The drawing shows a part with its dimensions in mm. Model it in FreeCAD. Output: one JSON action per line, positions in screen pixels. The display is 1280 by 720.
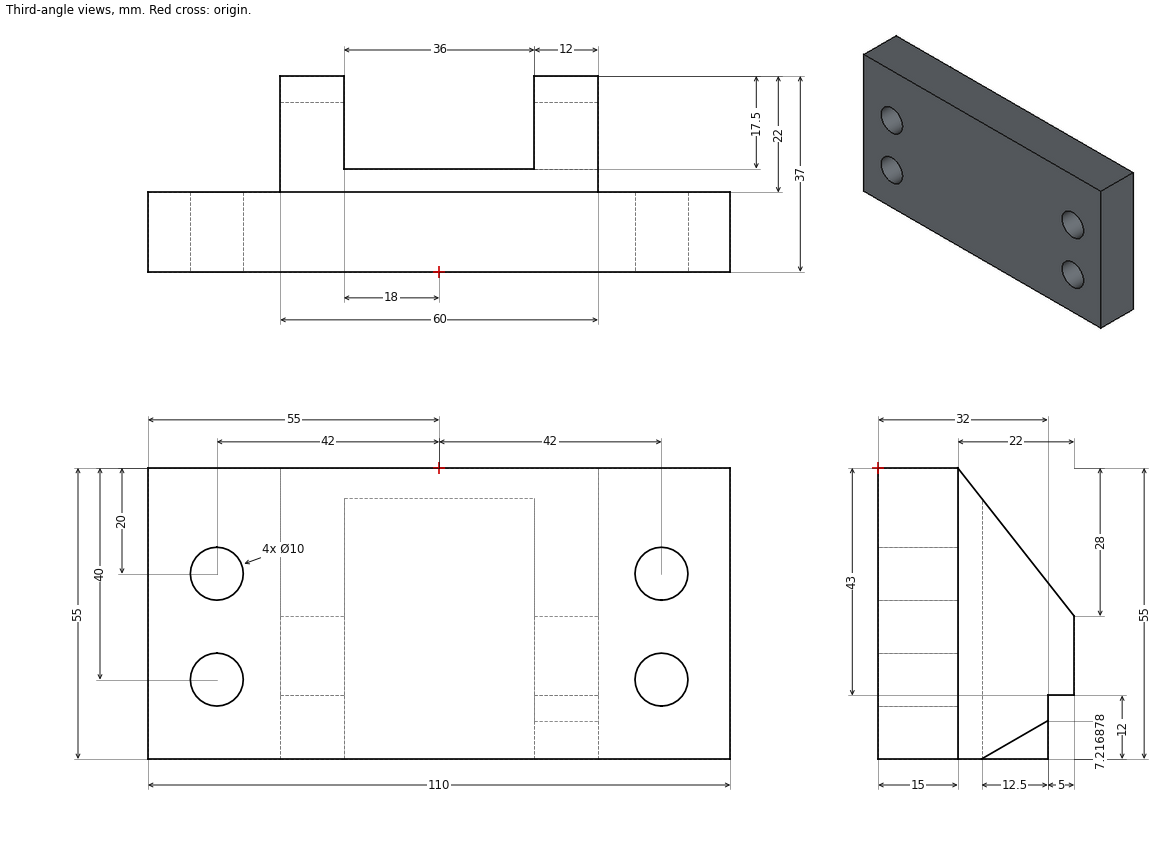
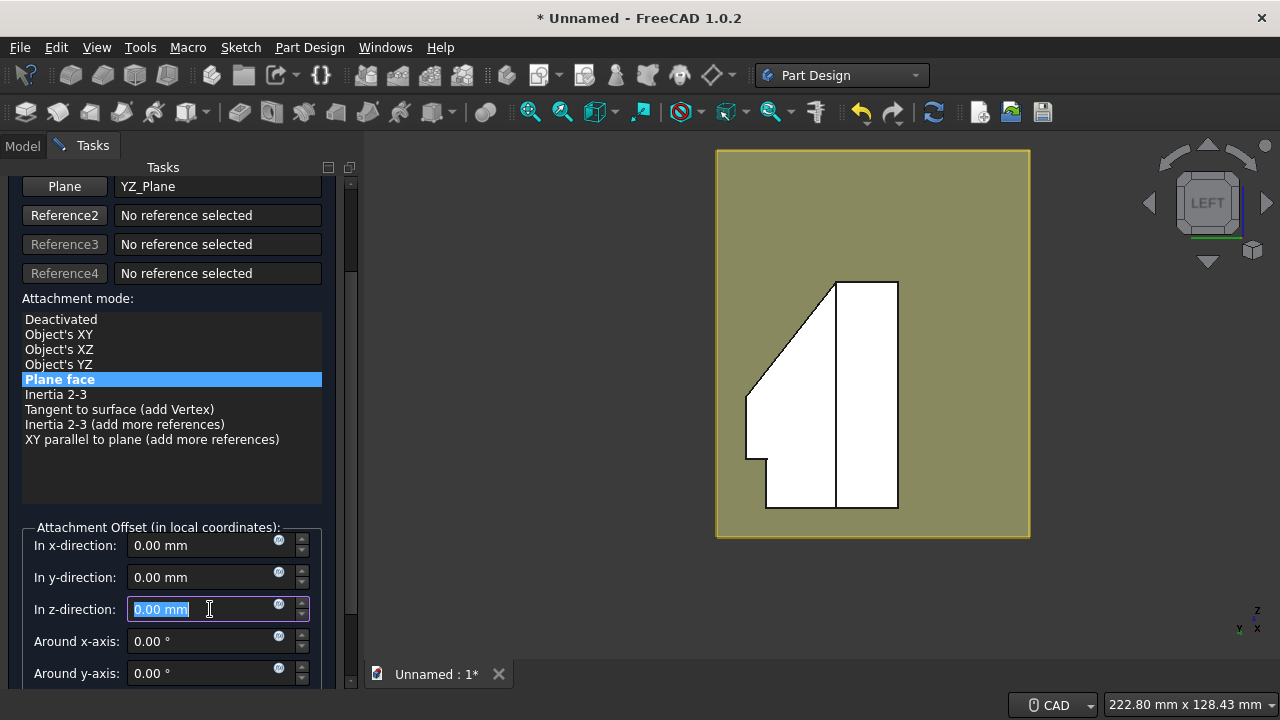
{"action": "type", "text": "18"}
{"action": "key", "text": "Tab"}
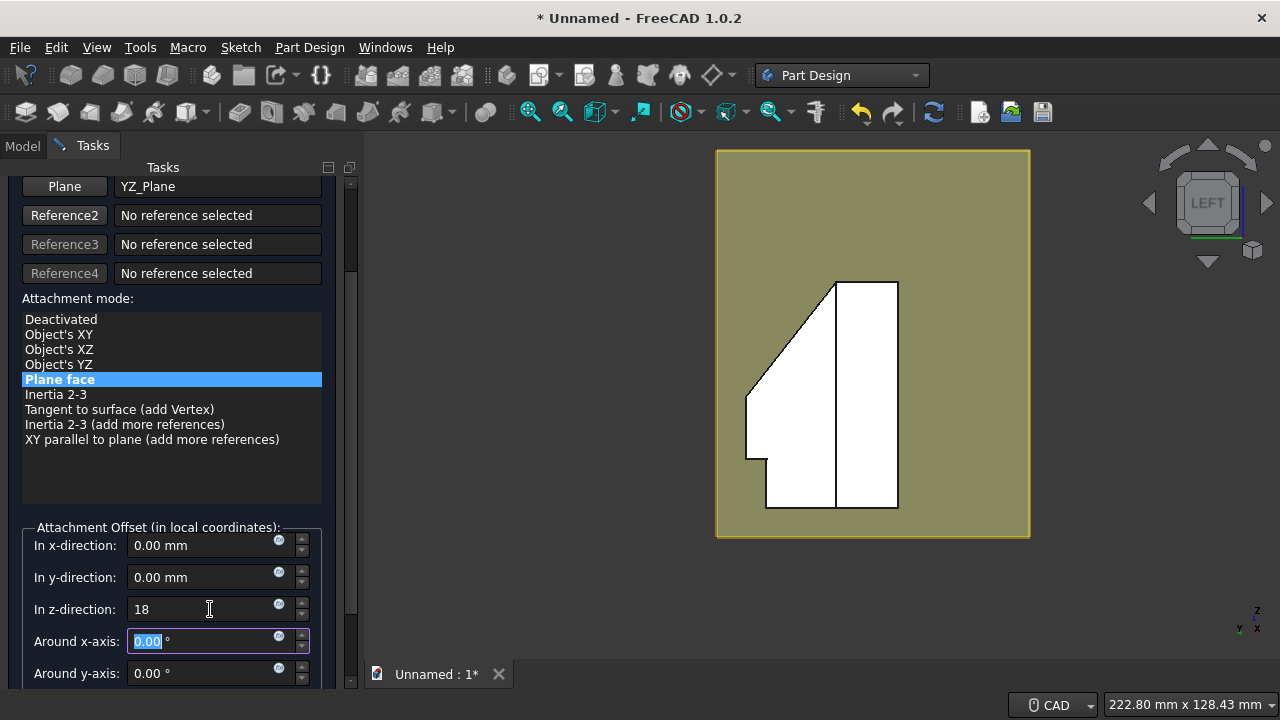
{"action": "scroll", "coordinate": [351, 432], "scroll_direction": "up", "scroll_amount": 3}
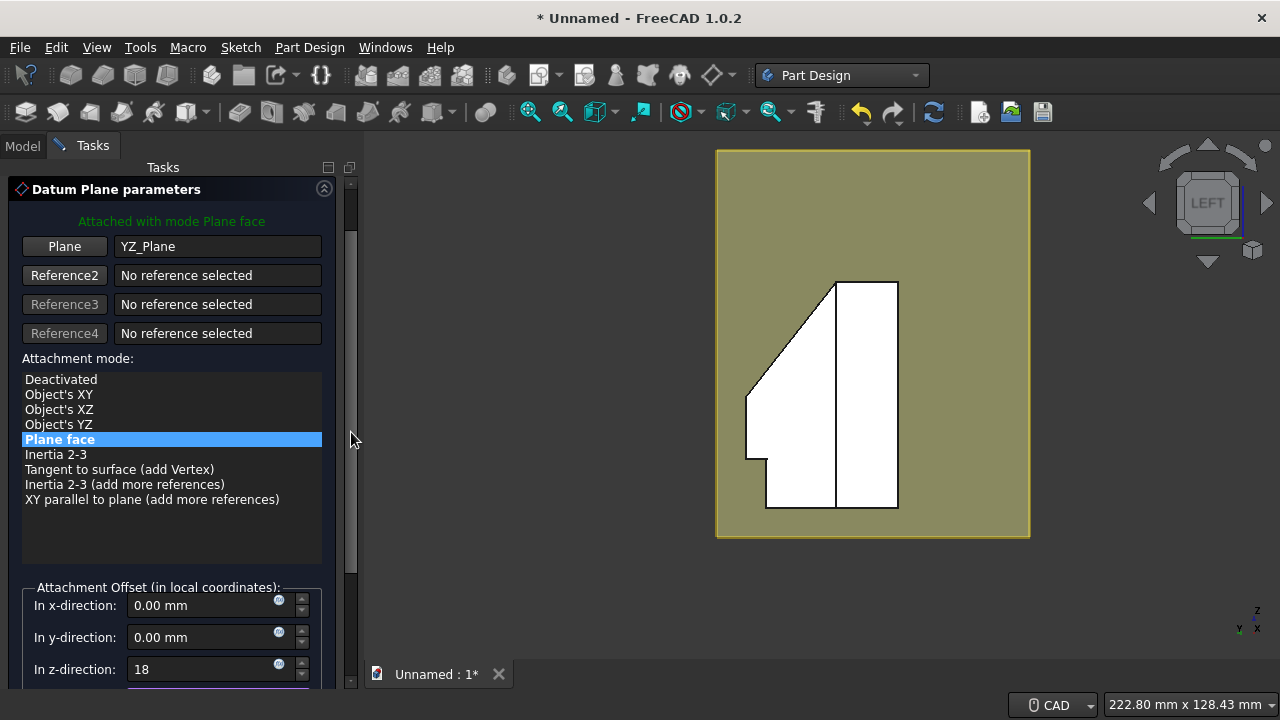
{"action": "left_click", "coordinate": [124, 206]}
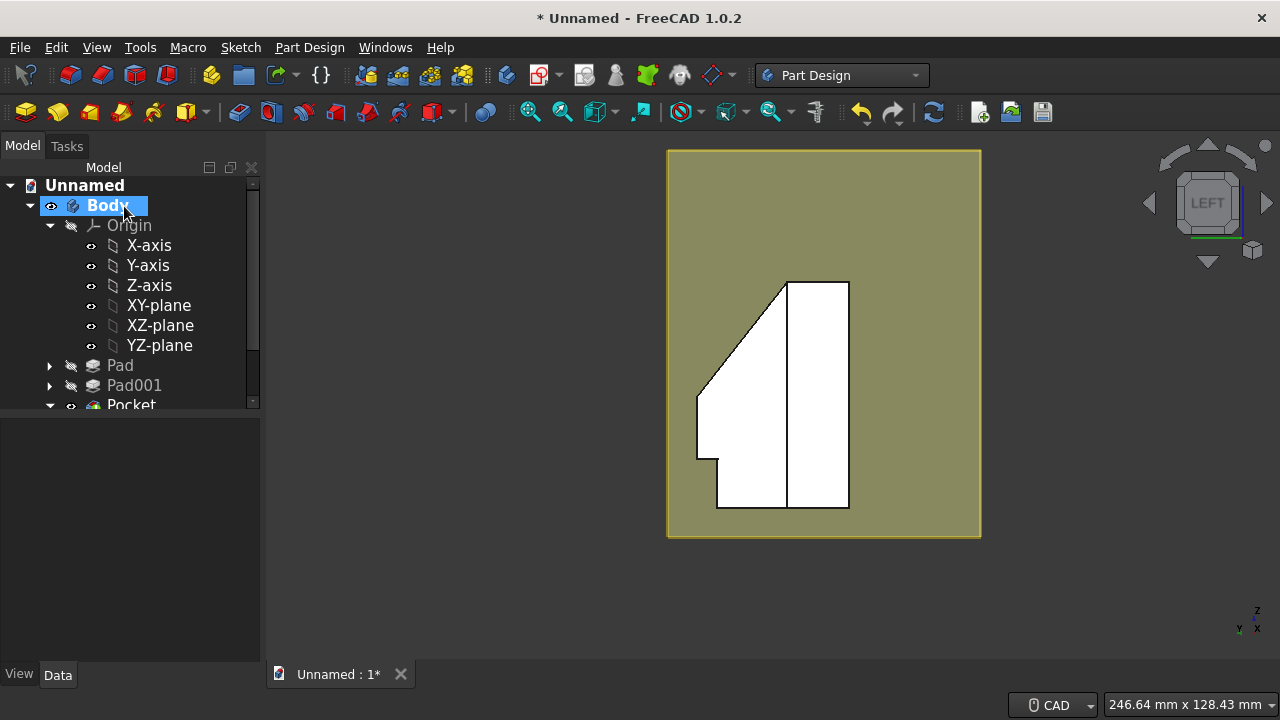
{"action": "scroll", "coordinate": [100, 301], "scroll_direction": "down", "scroll_amount": 3}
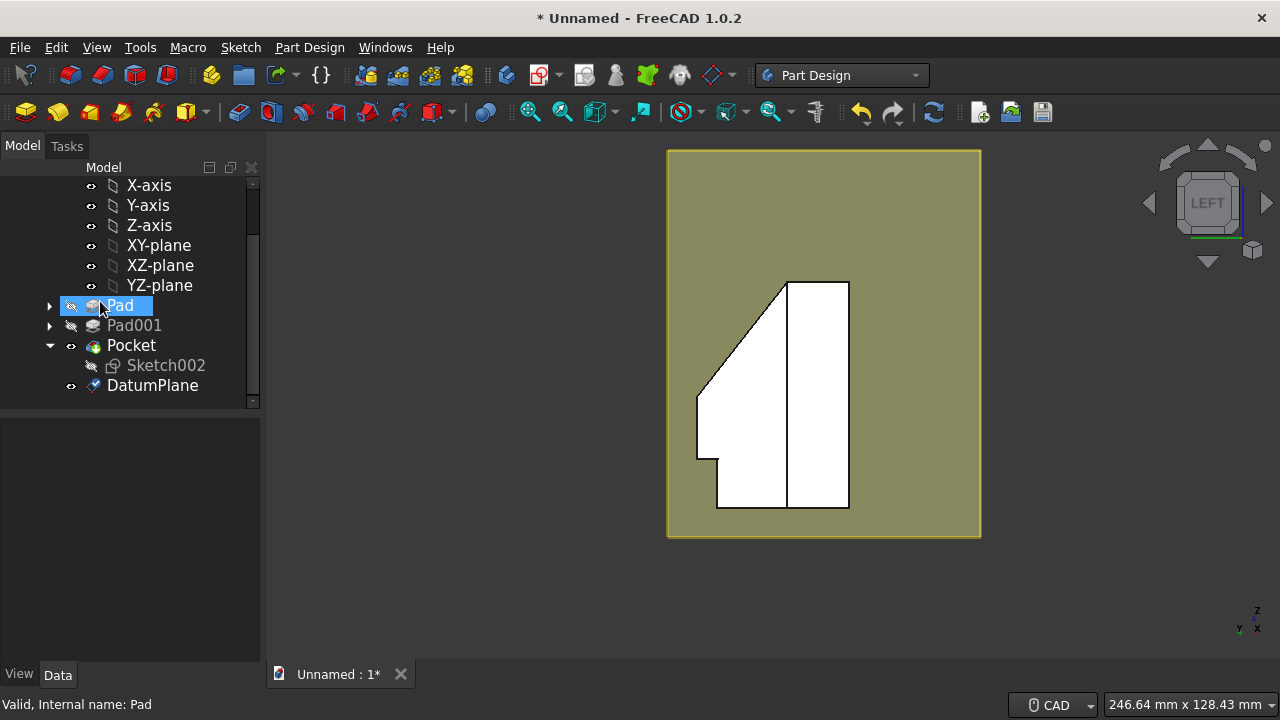
{"action": "left_click", "coordinate": [116, 386]}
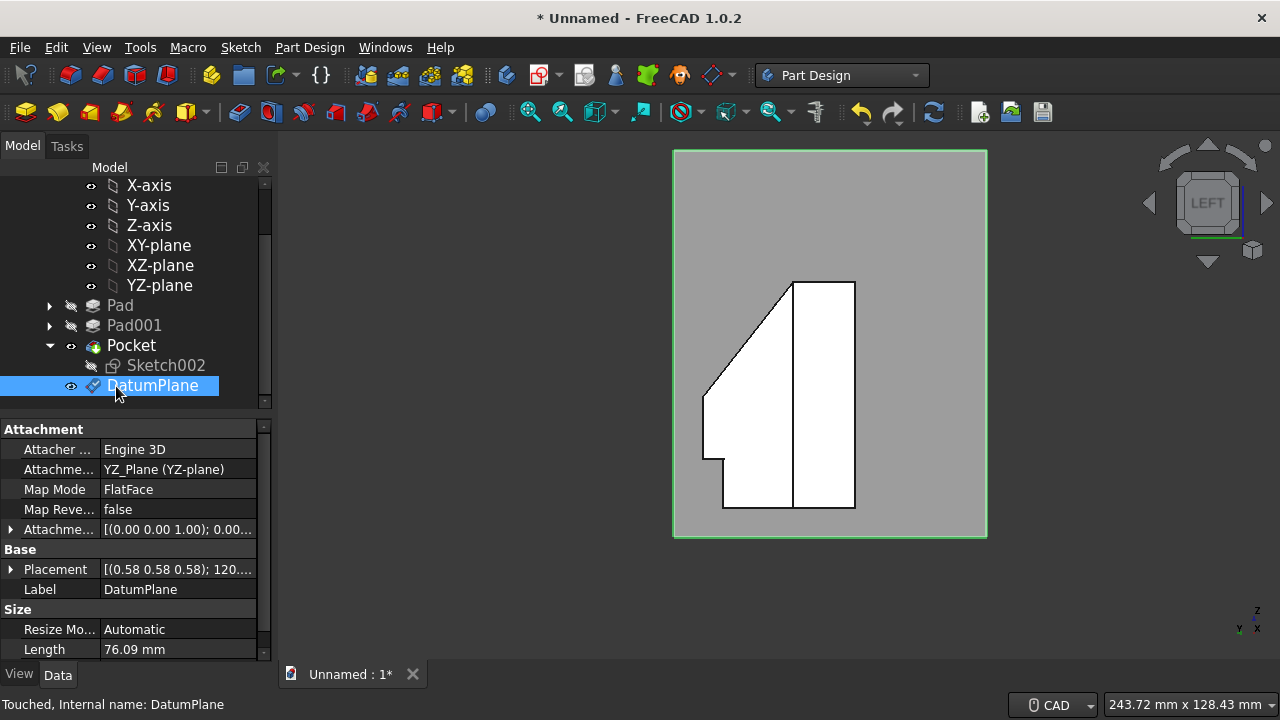
{"action": "left_click", "coordinate": [540, 76]}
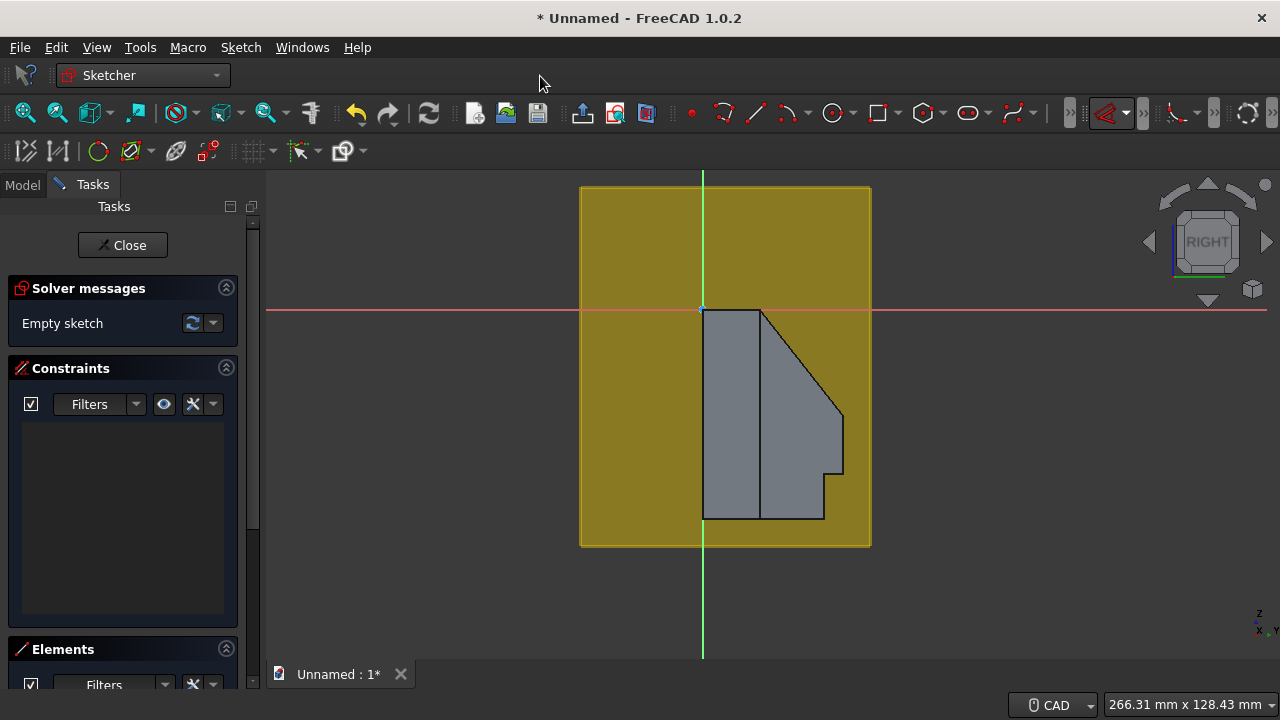
{"action": "left_click", "coordinate": [648, 114]}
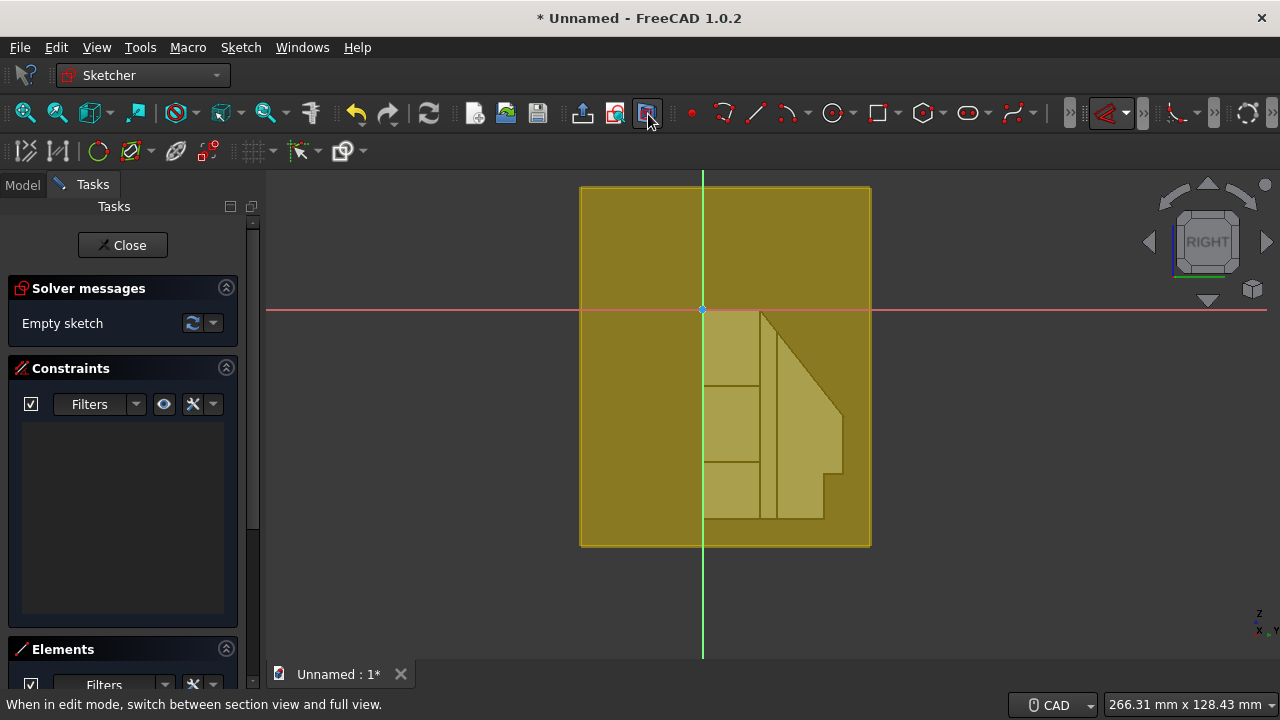
{"action": "scroll", "coordinate": [810, 515], "scroll_direction": "up", "scroll_amount": 12}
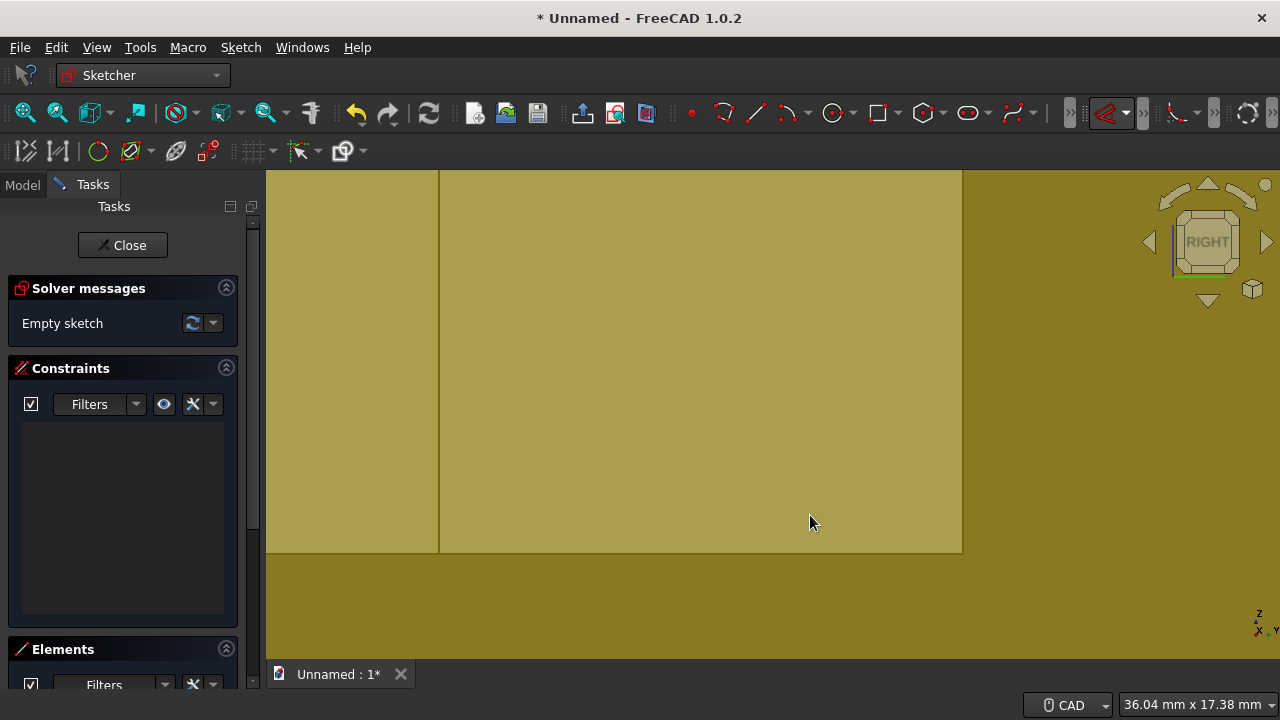
{"action": "left_click", "coordinate": [724, 114]}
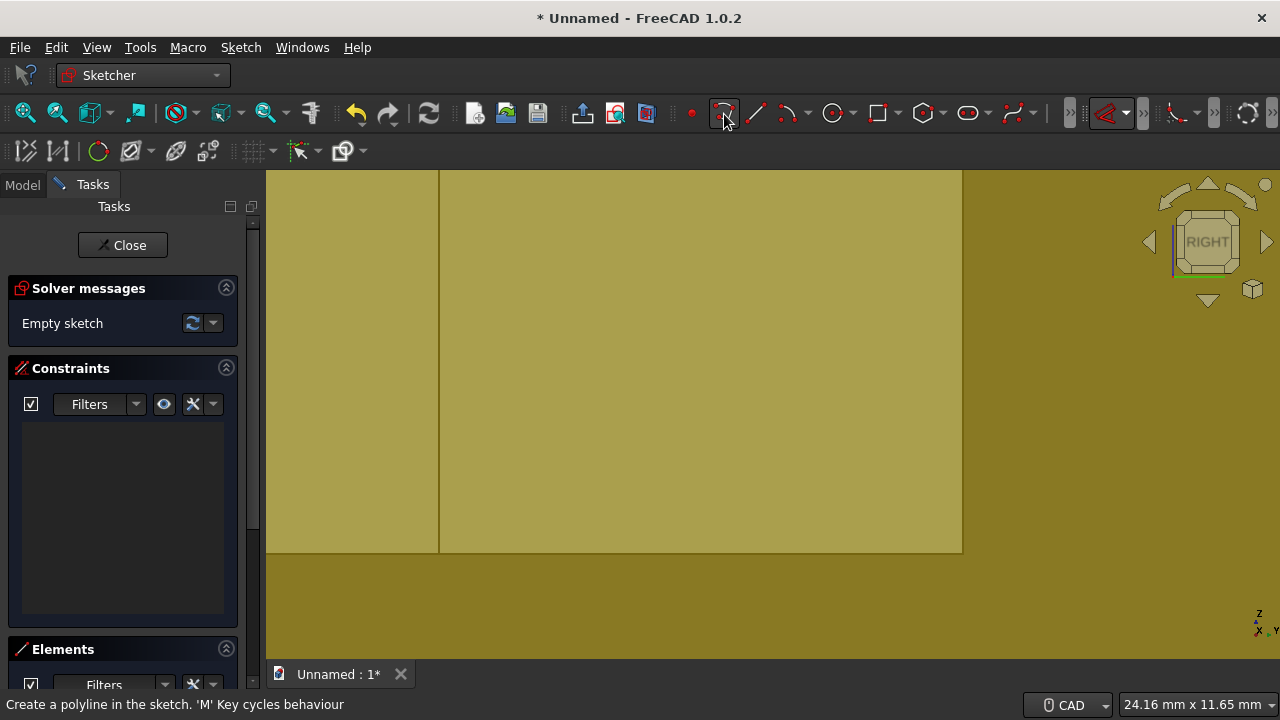
{"action": "left_click", "coordinate": [963, 251]}
{"action": "left_click", "coordinate": [963, 554]}
{"action": "left_click", "coordinate": [439, 554]}
{"action": "left_click", "coordinate": [963, 252]}
{"action": "key", "text": "Escape"}
{"action": "key", "text": "Escape"}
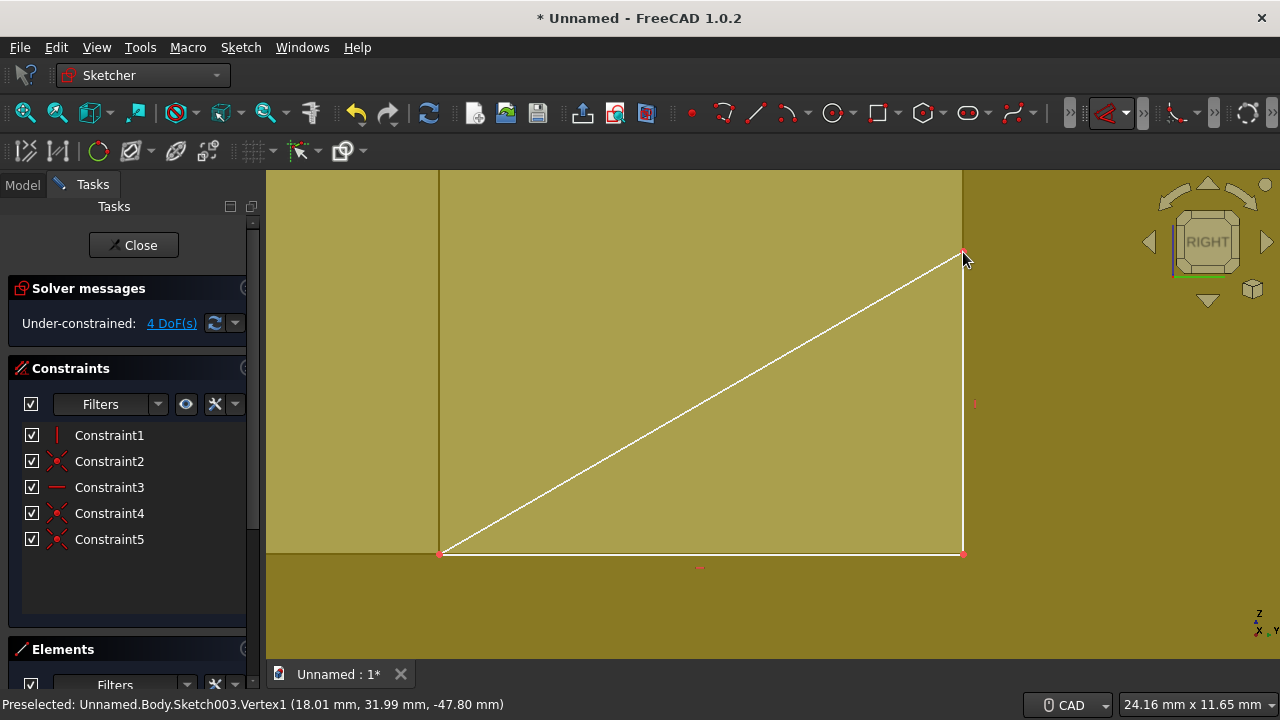
{"action": "left_click", "coordinate": [963, 252]}